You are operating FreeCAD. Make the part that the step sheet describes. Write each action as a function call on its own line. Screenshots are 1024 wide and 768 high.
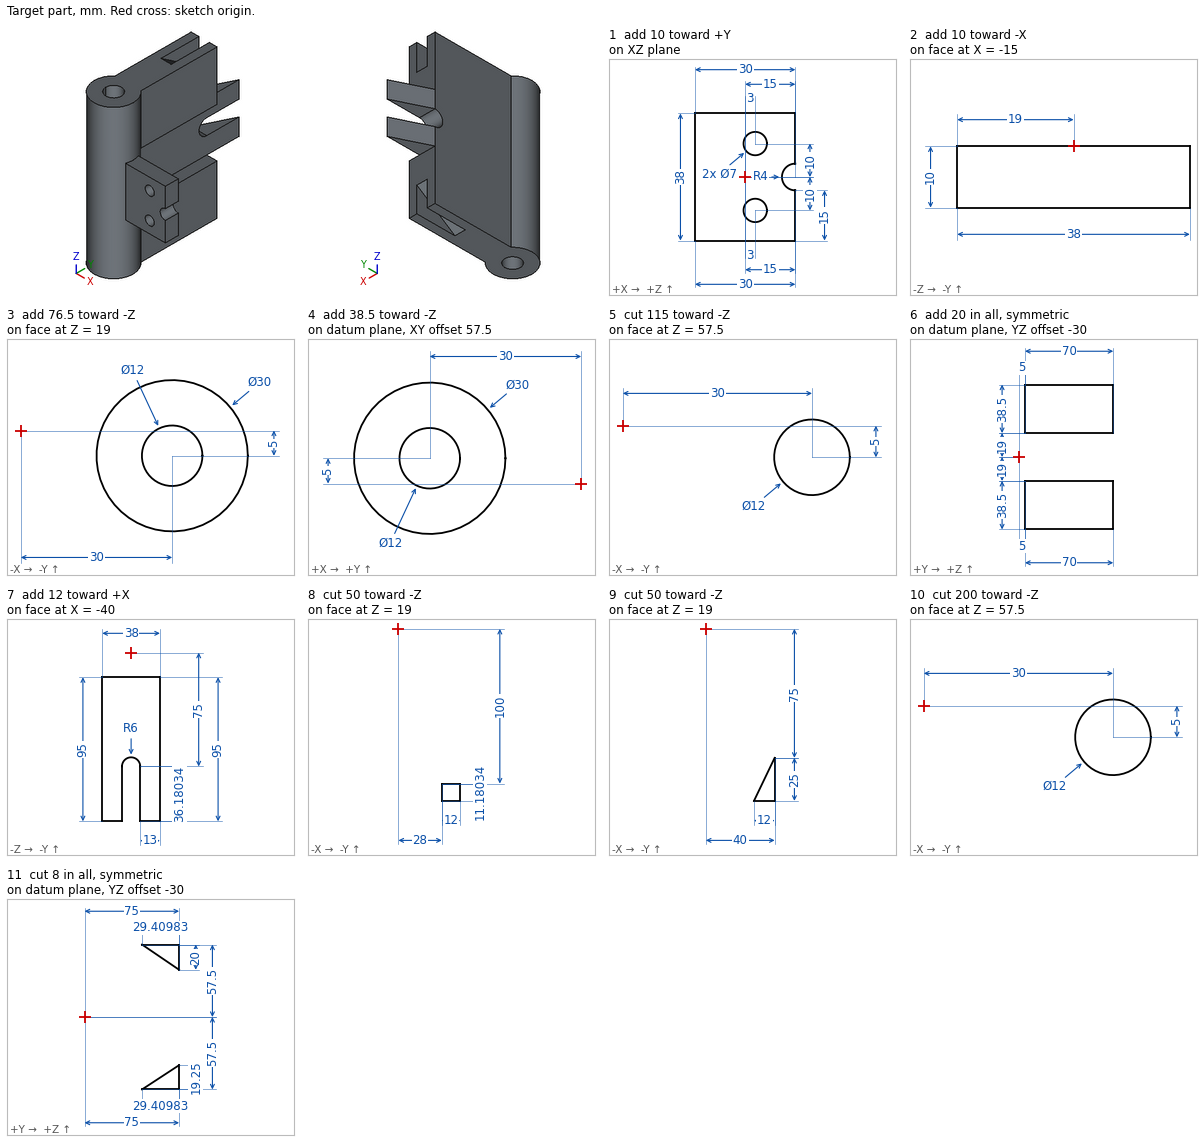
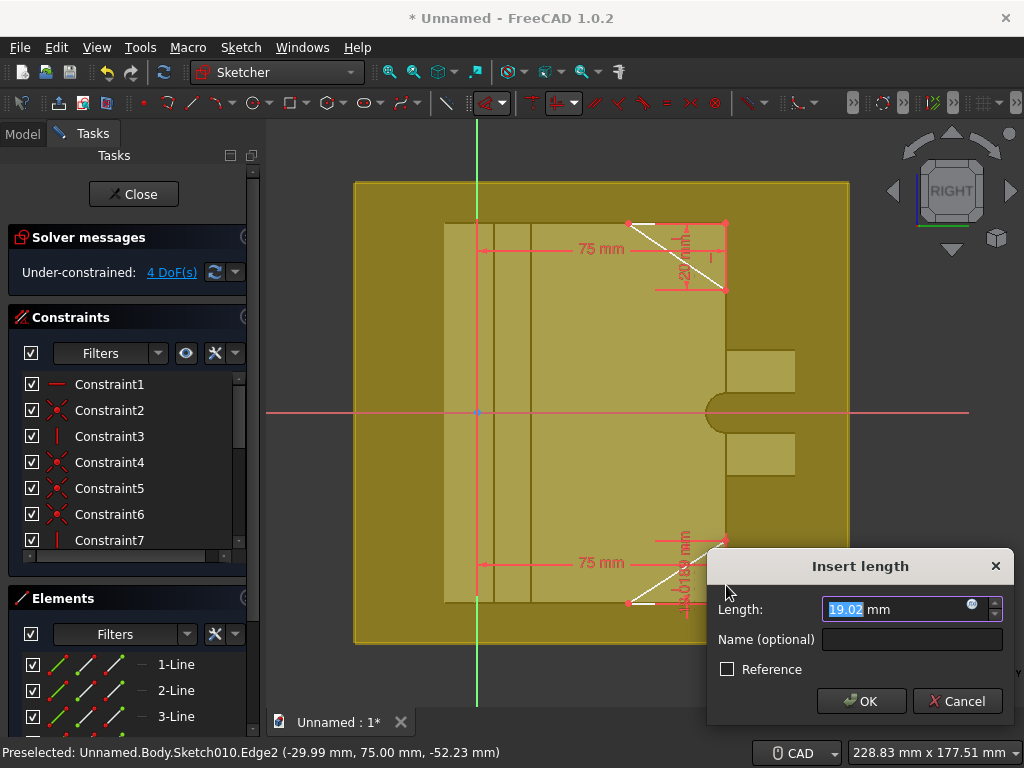
text(19.25)
key(Return)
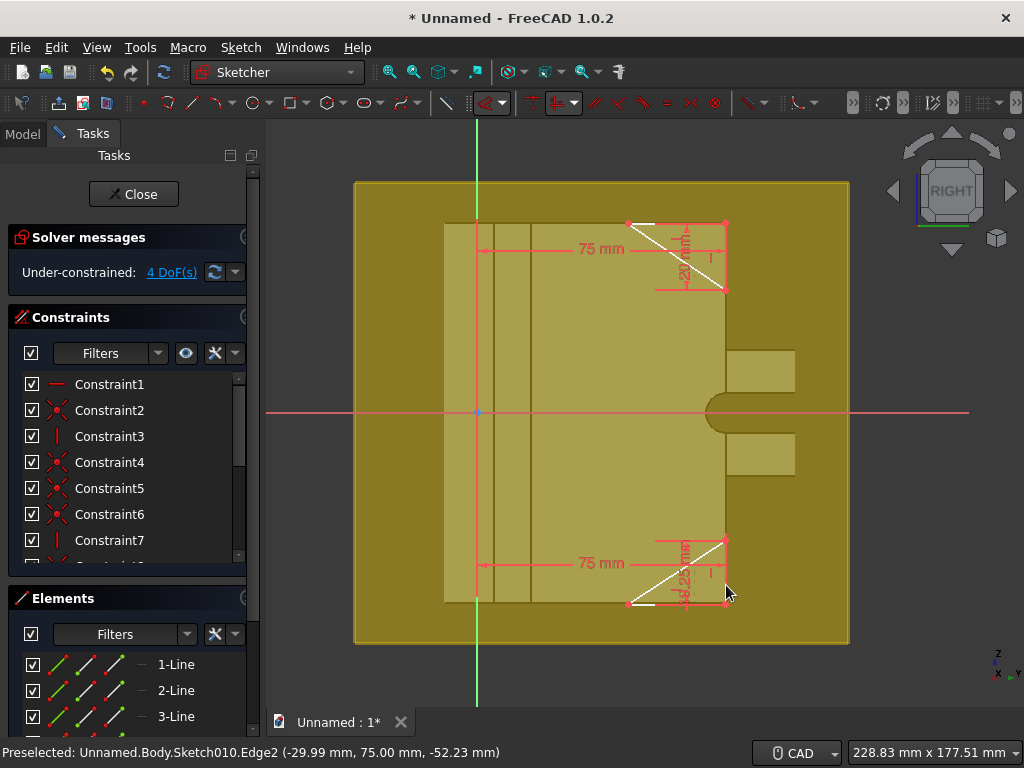
click(628, 605)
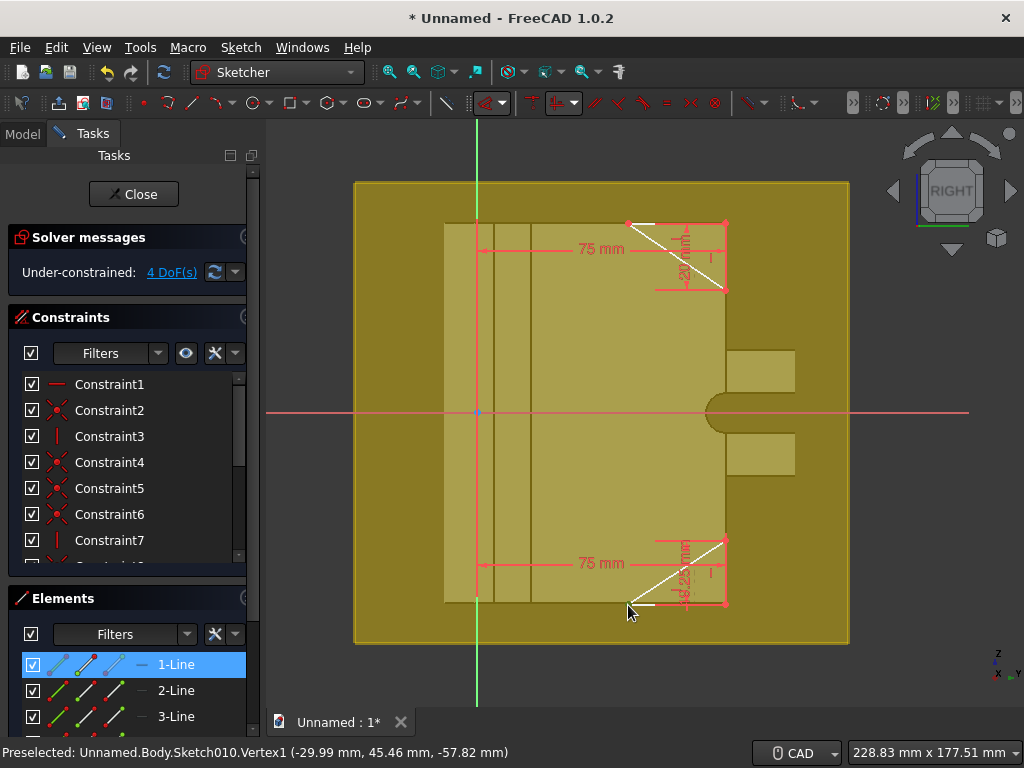
click(504, 104)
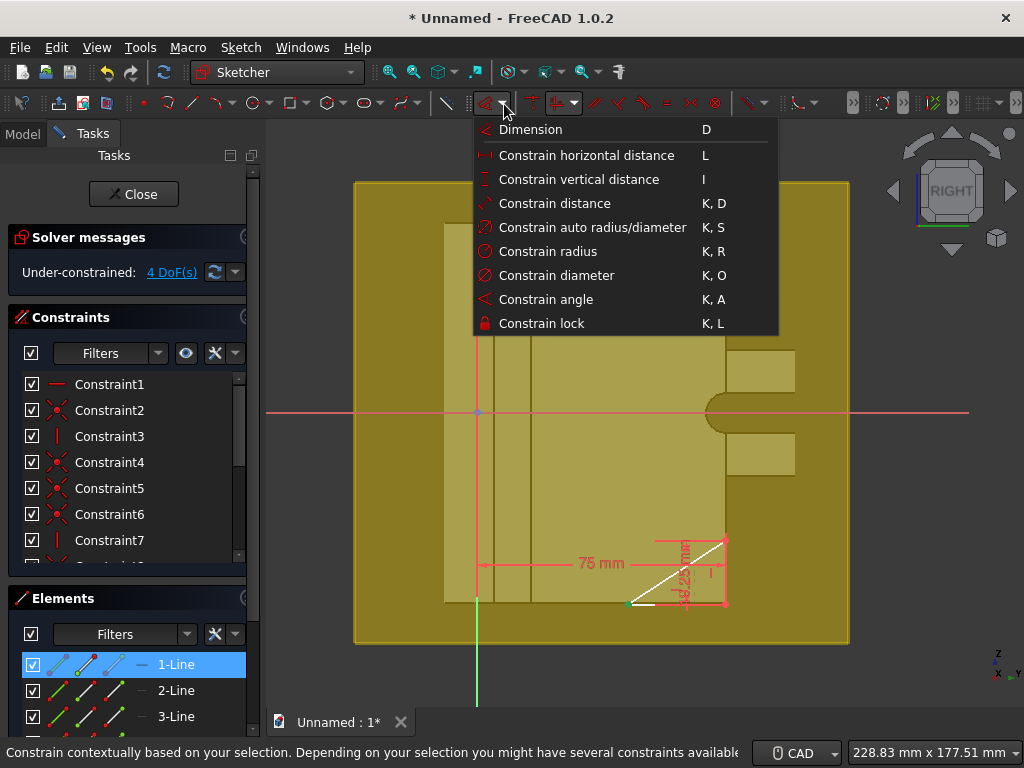
click(626, 179)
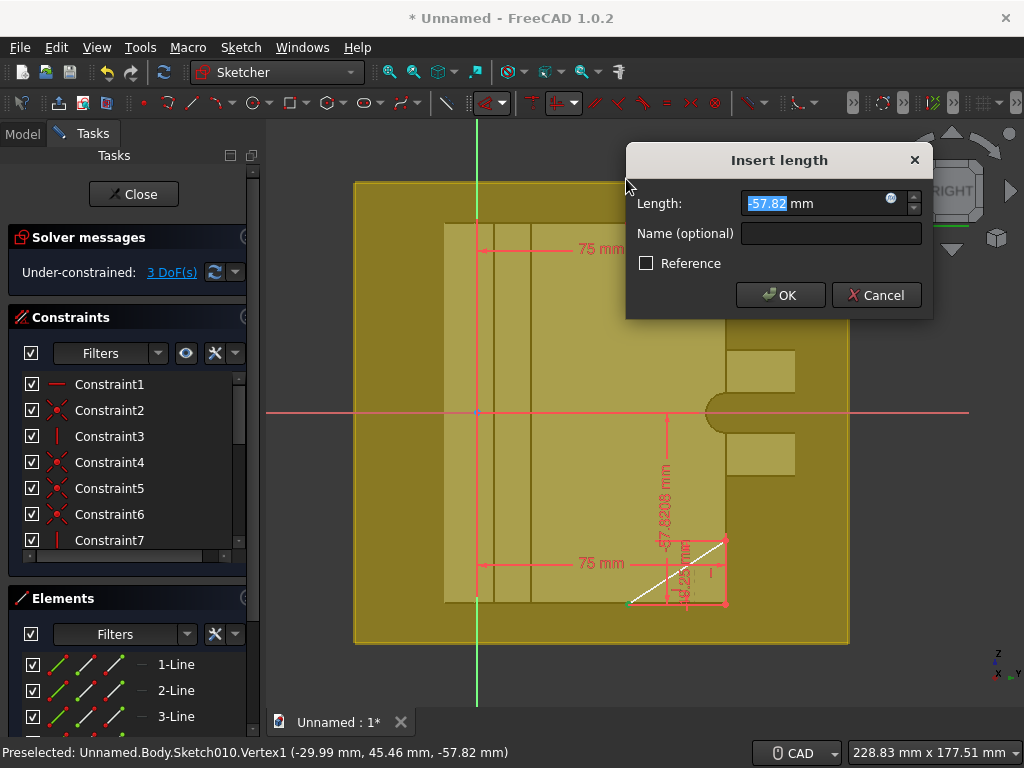
text(-57.5)
key(Return)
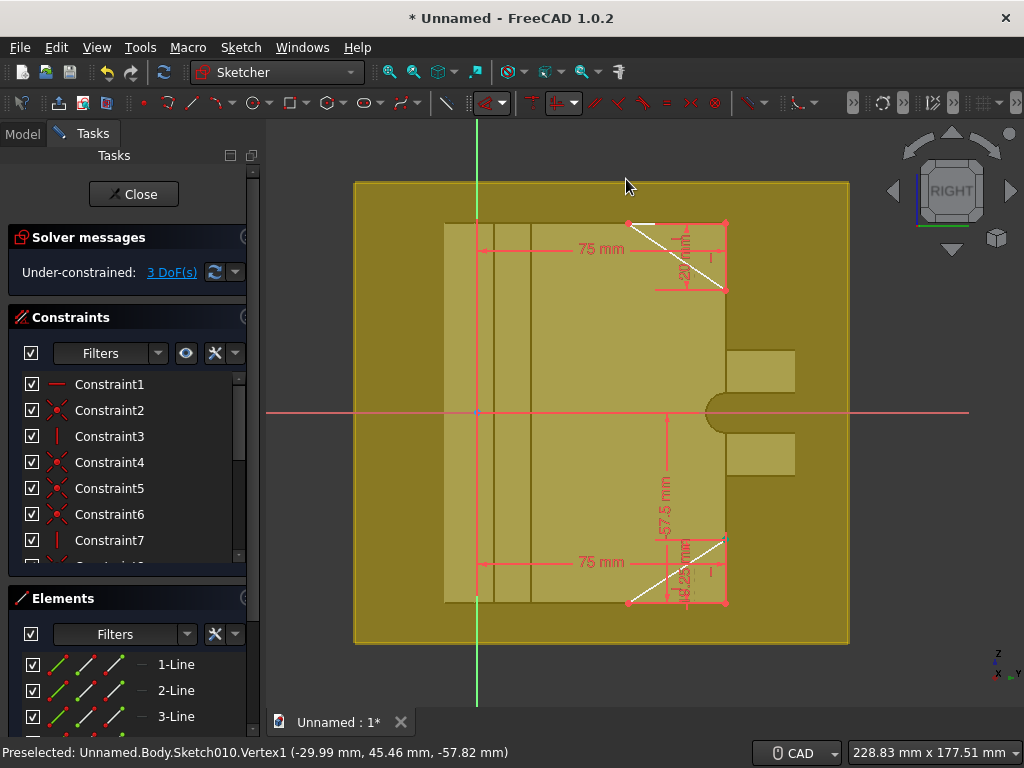
click(628, 224)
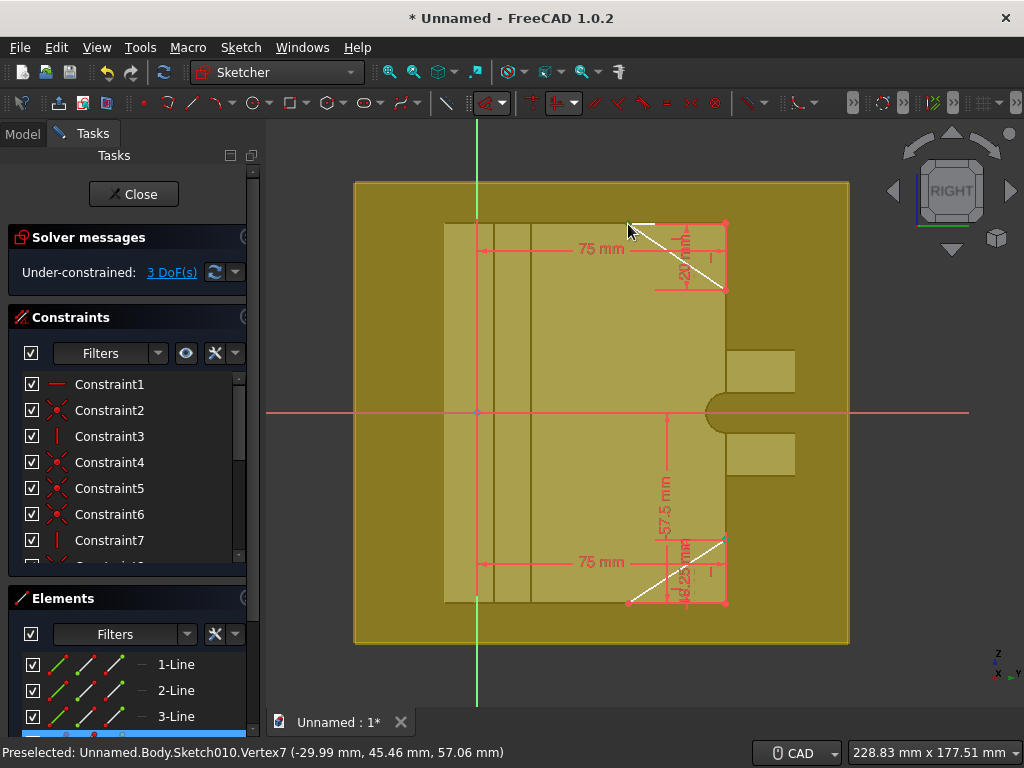
key(i)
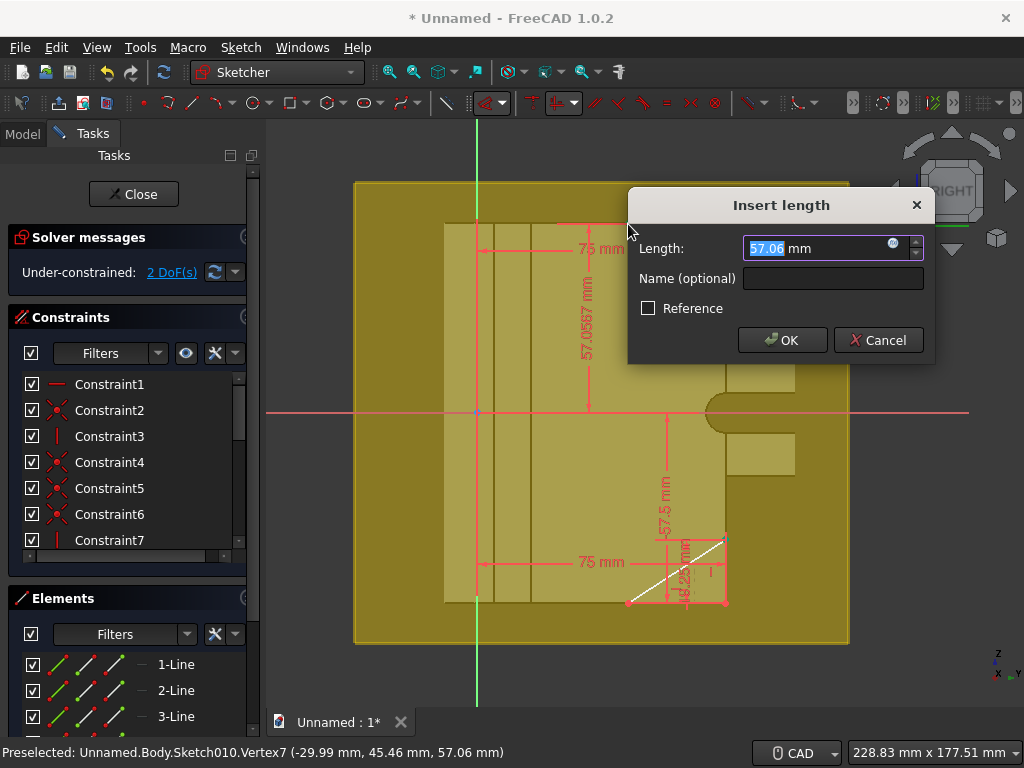
text(57.5)
key(Return)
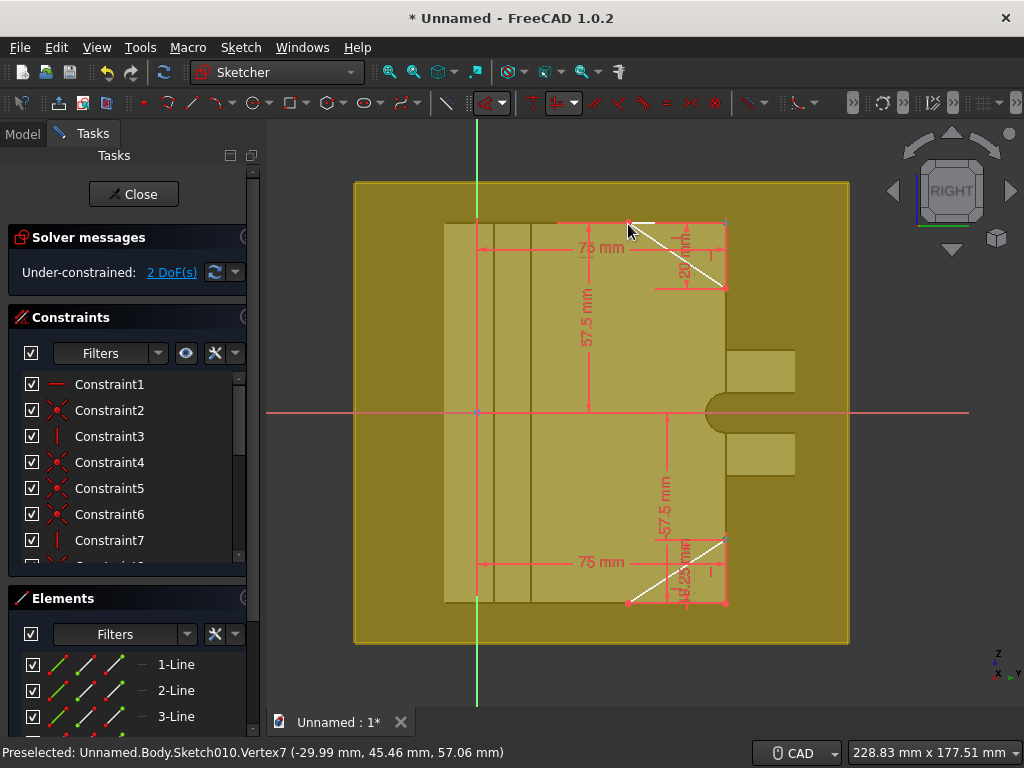
click(657, 603)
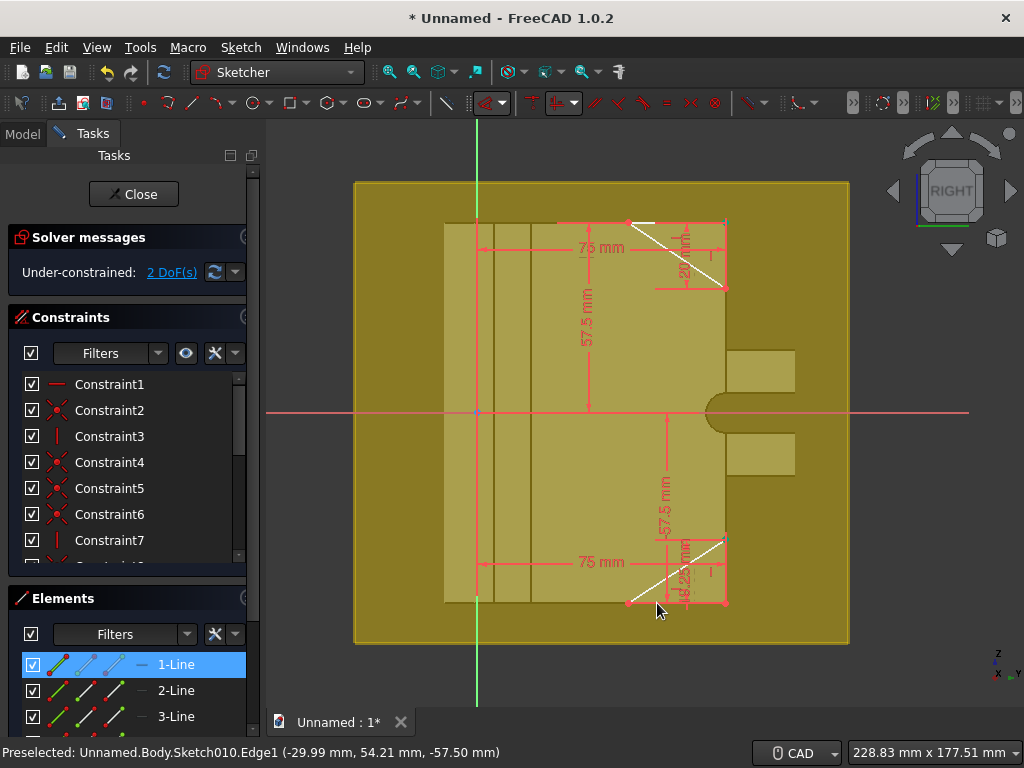
click(504, 104)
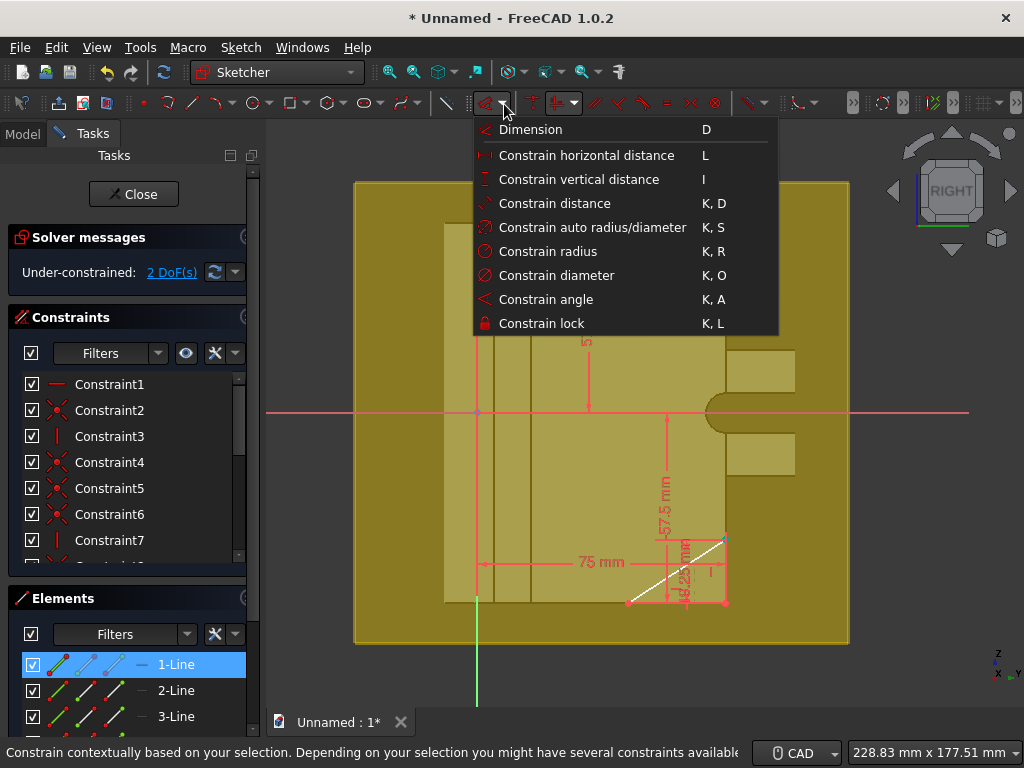
click(626, 155)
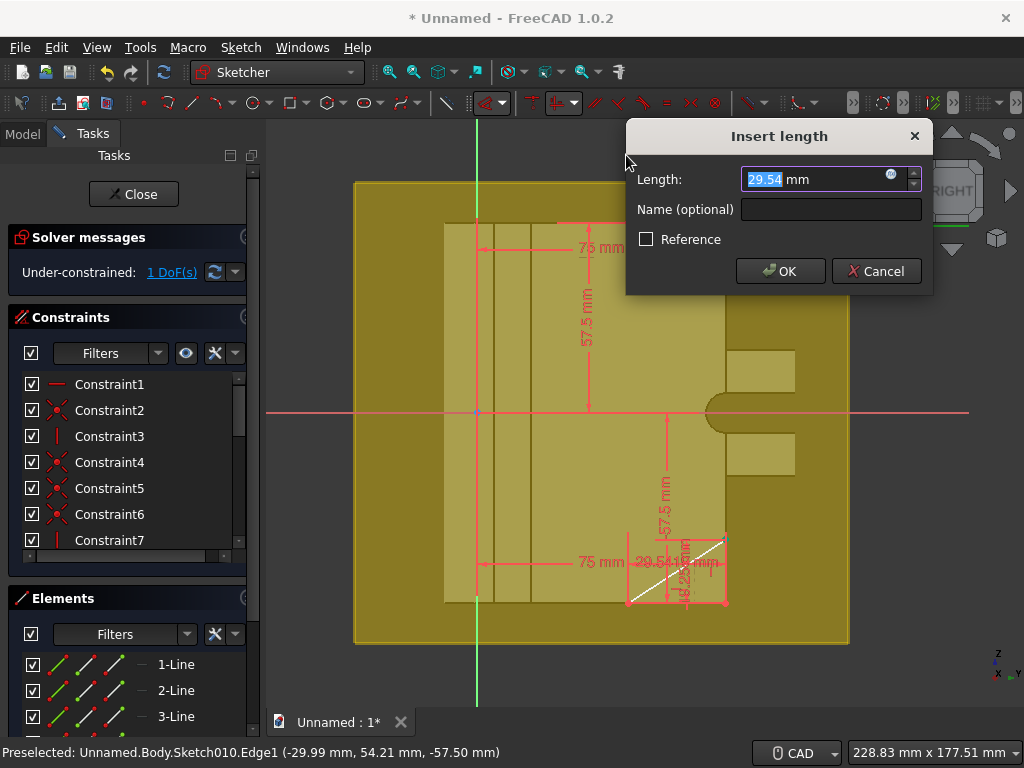
text(29.40983)
key(Return)